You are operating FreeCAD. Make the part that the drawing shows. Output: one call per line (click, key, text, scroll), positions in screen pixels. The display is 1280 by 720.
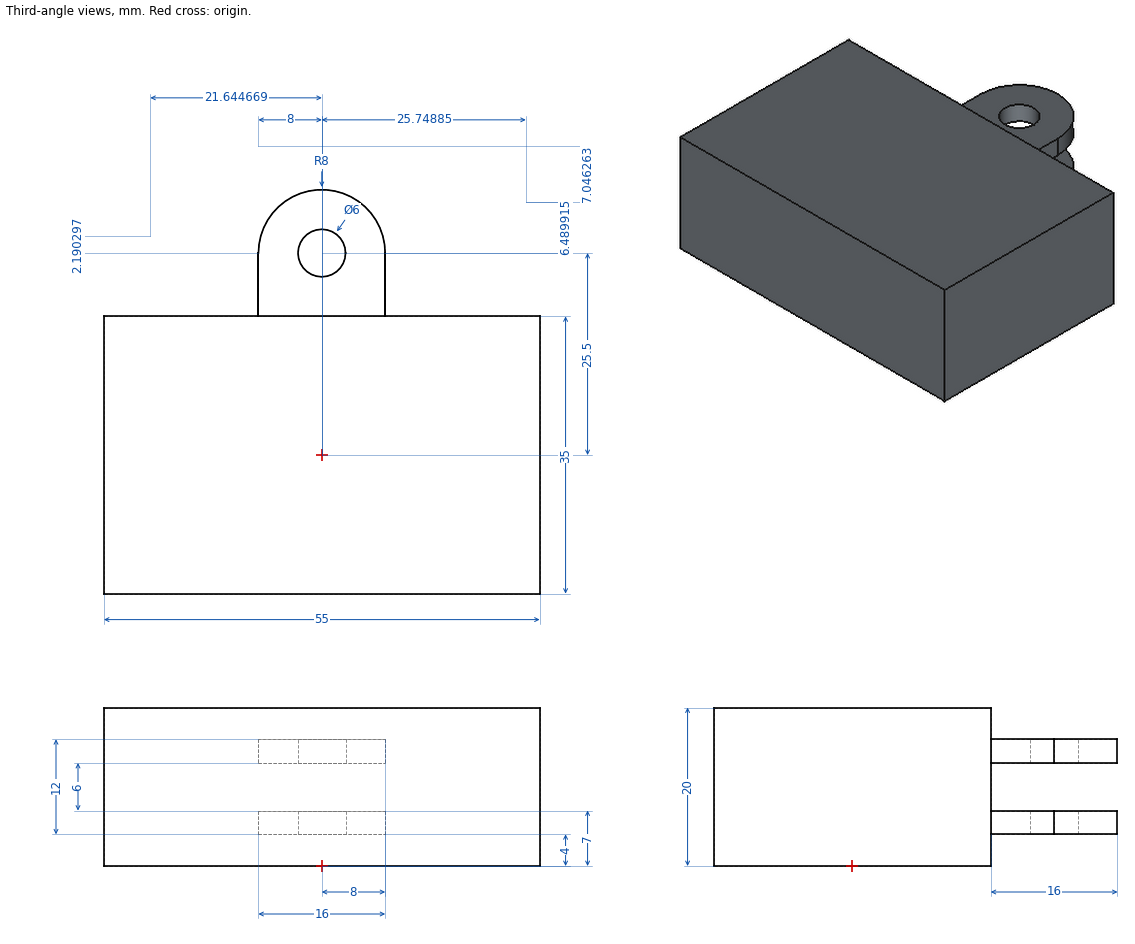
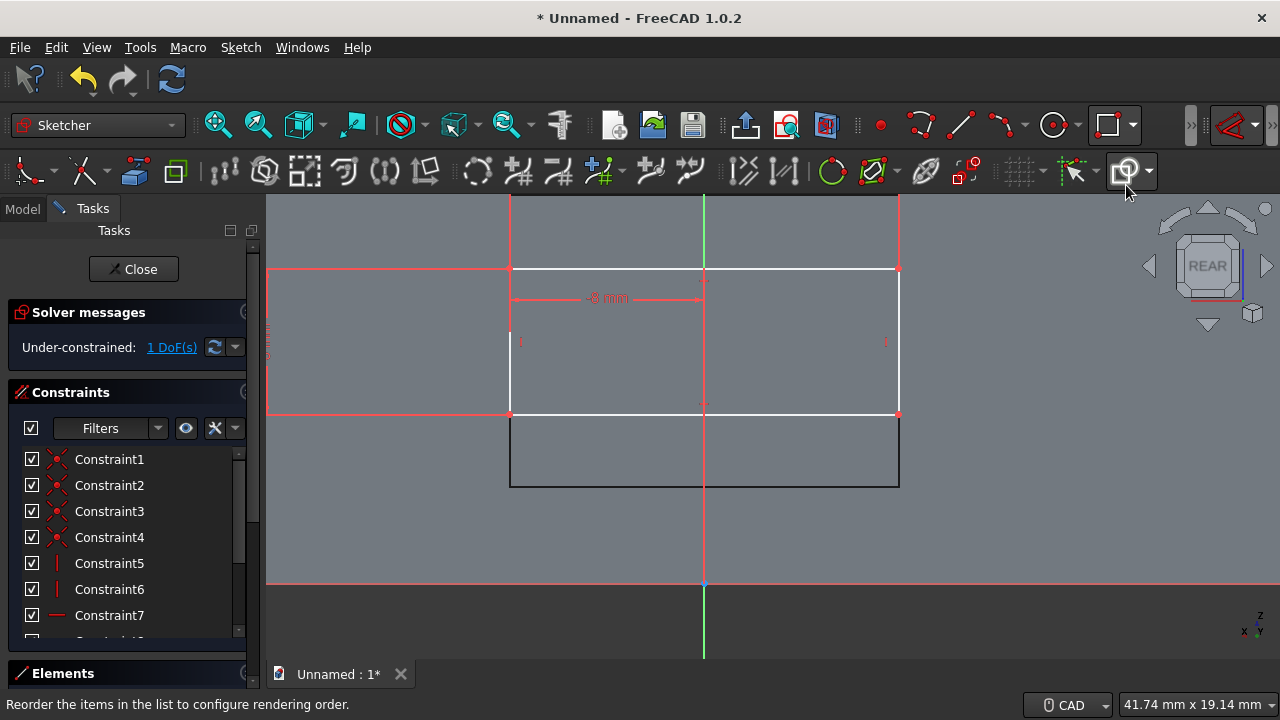
click(510, 415)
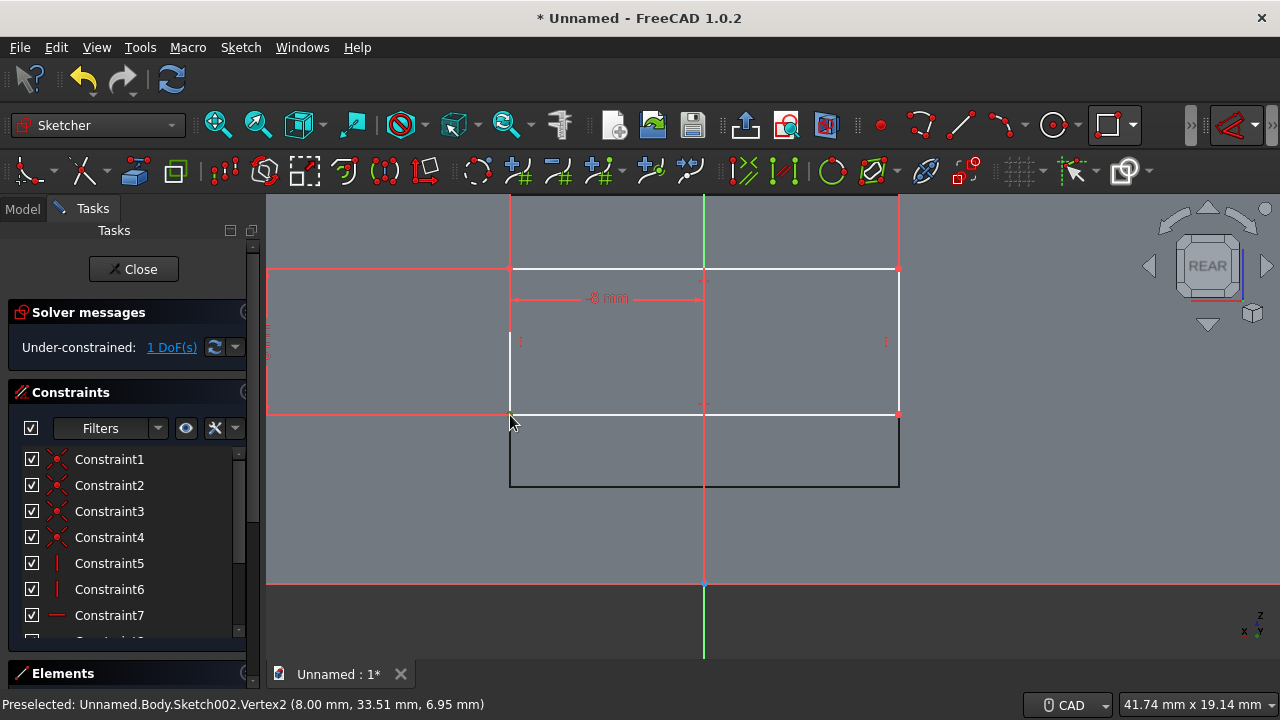
click(1258, 126)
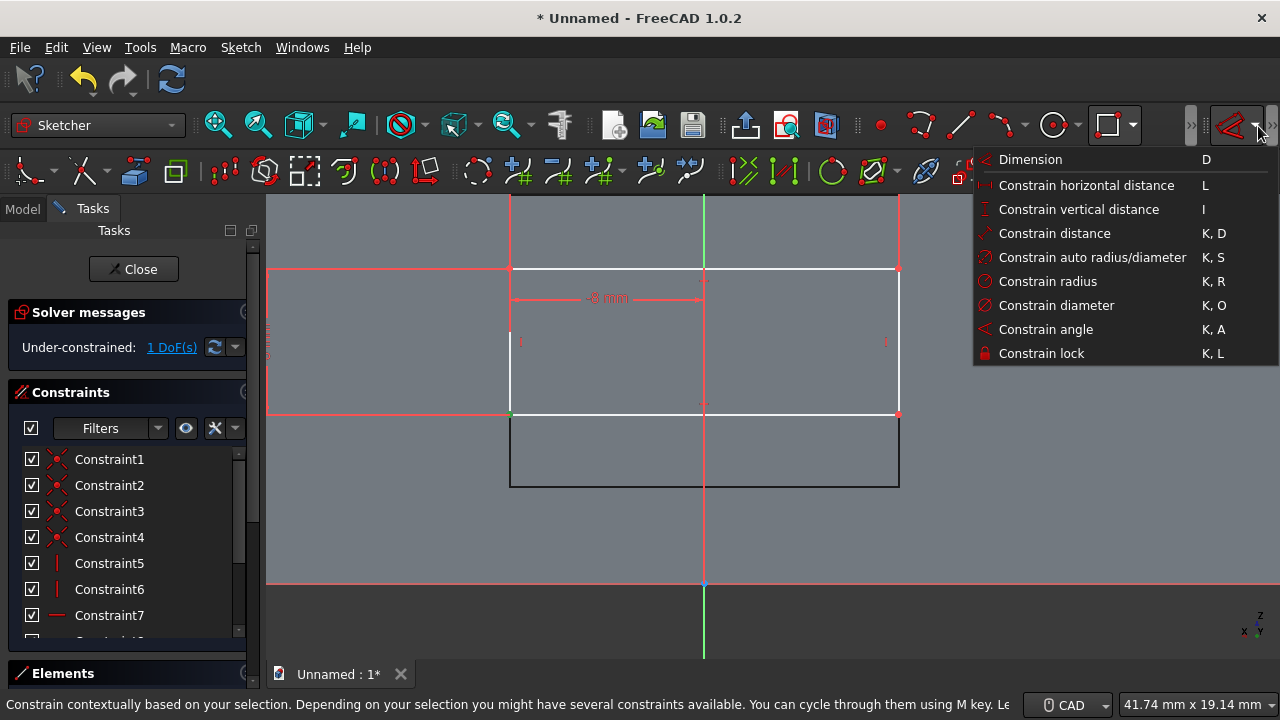
click(1126, 209)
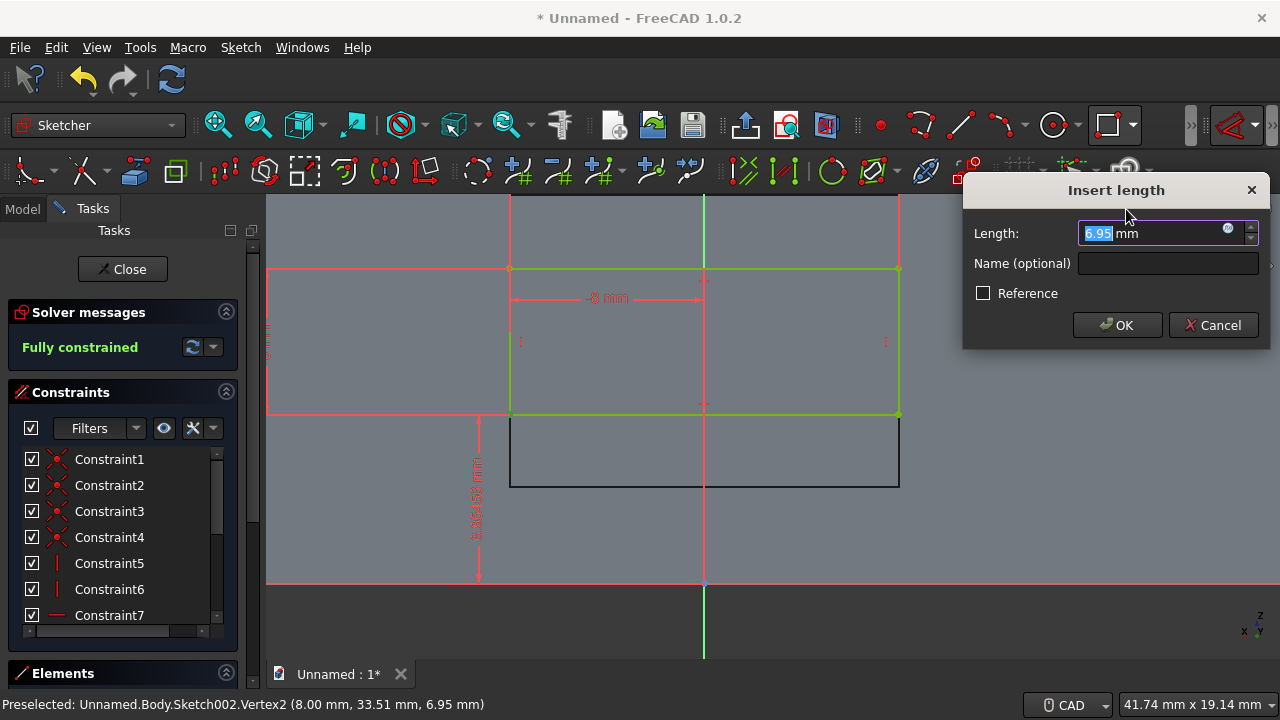
text(7)
key(Return)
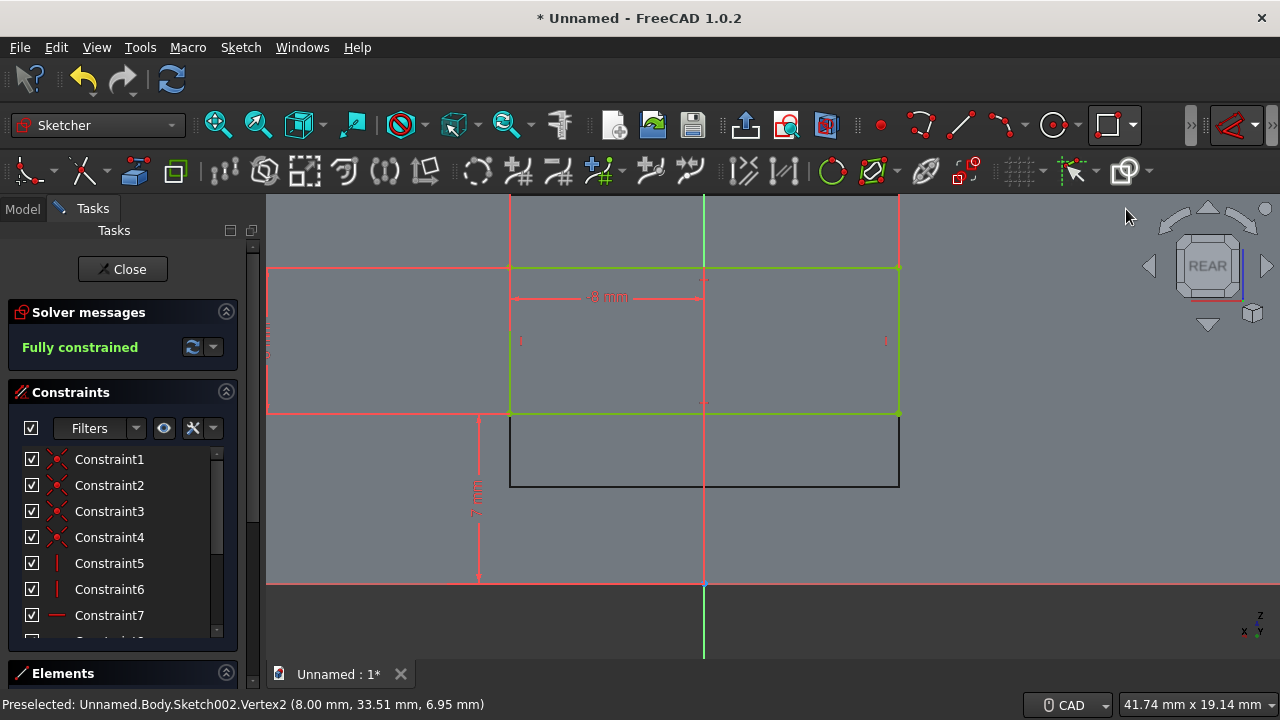
click(123, 269)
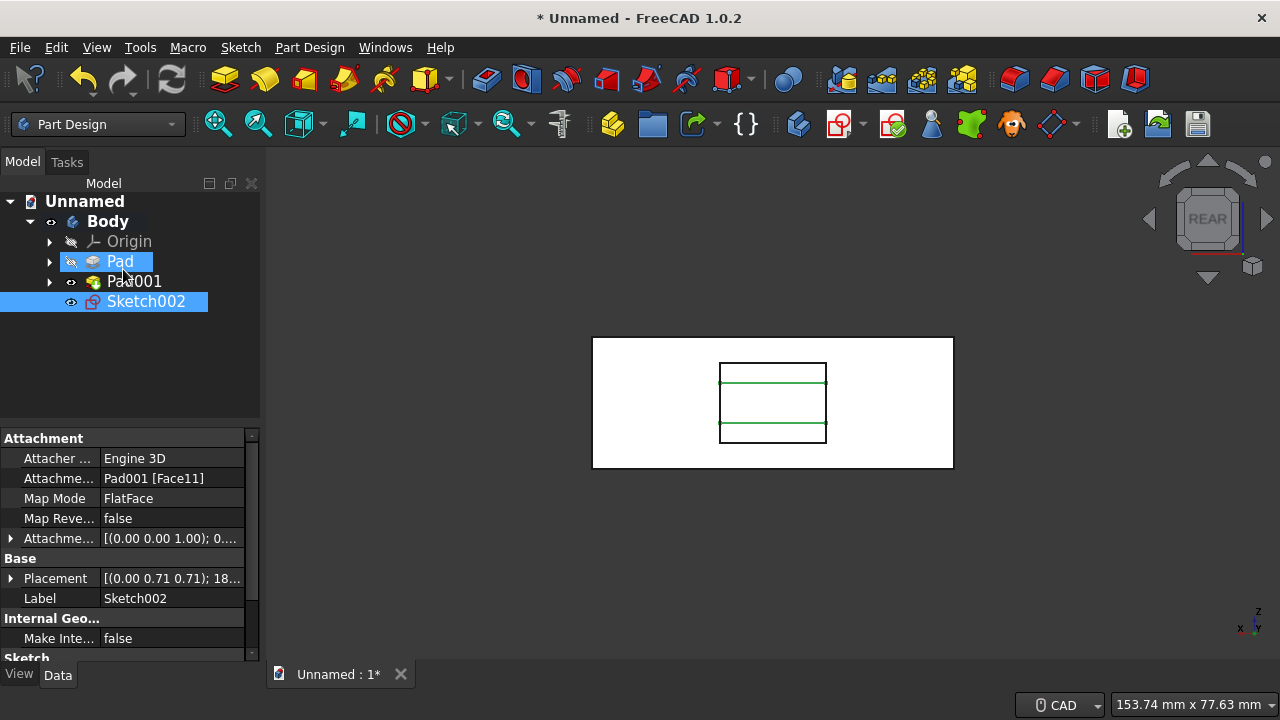
click(488, 80)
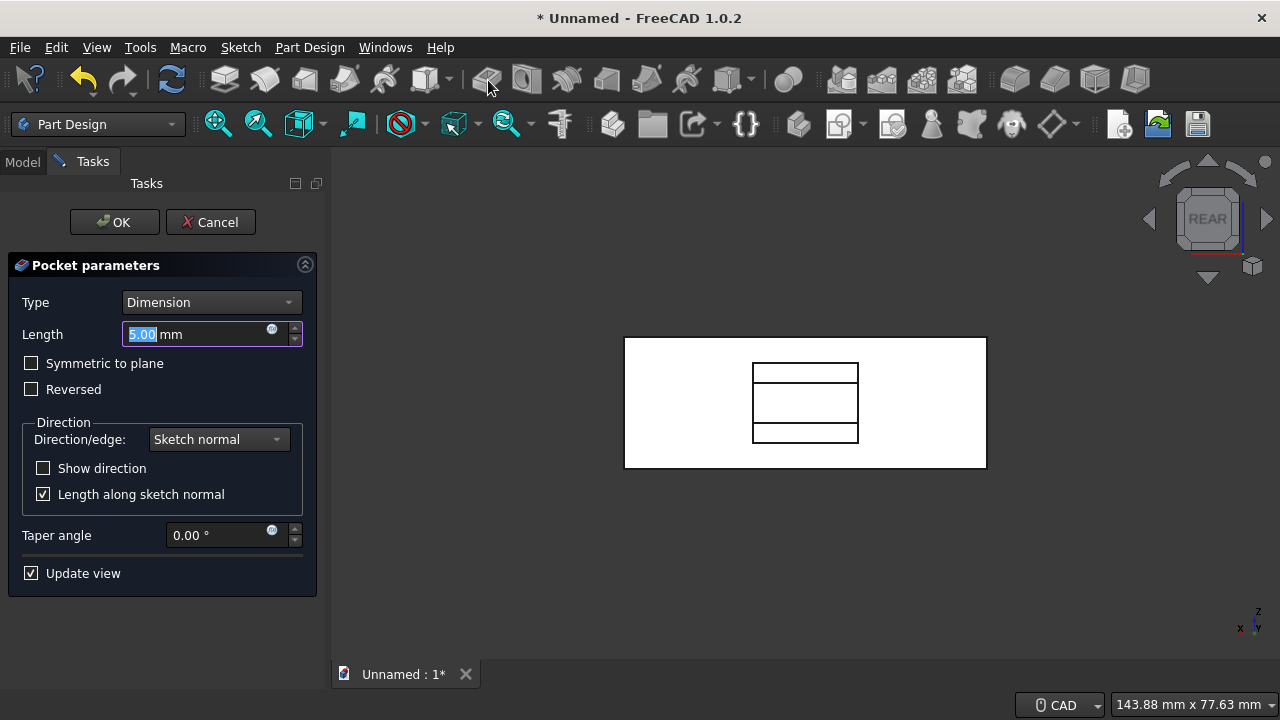
click(212, 302)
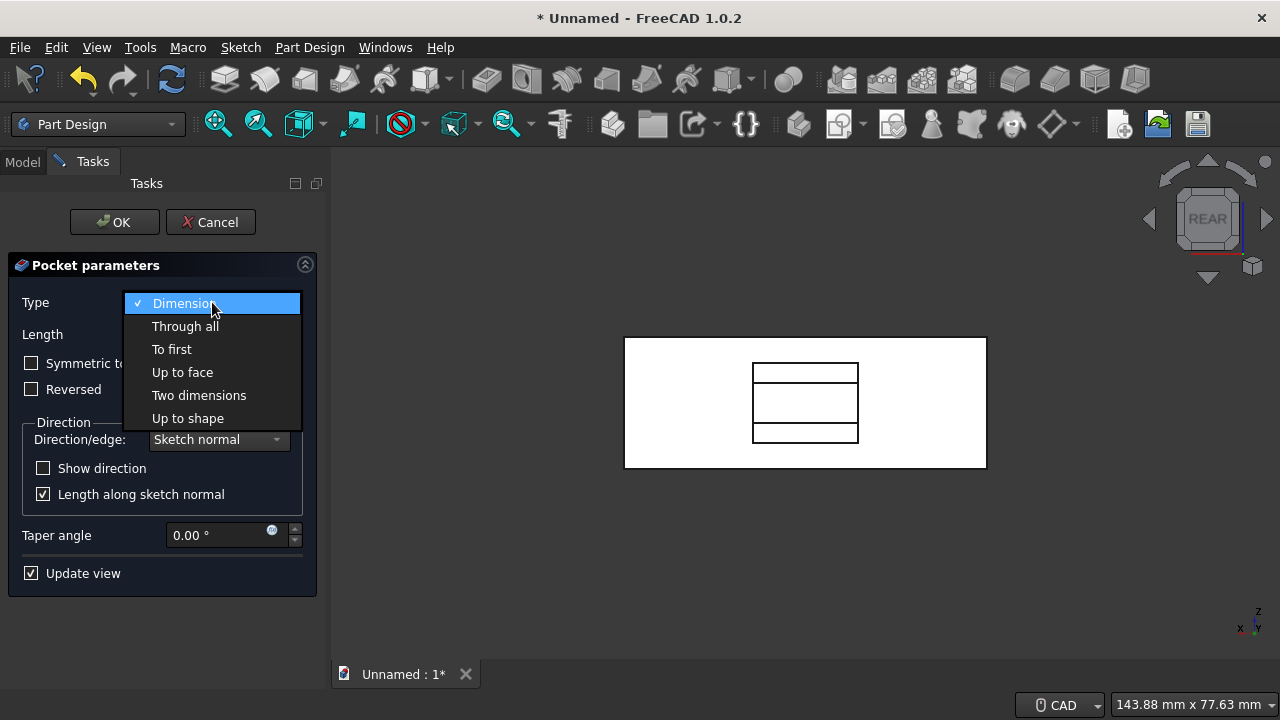
click(212, 396)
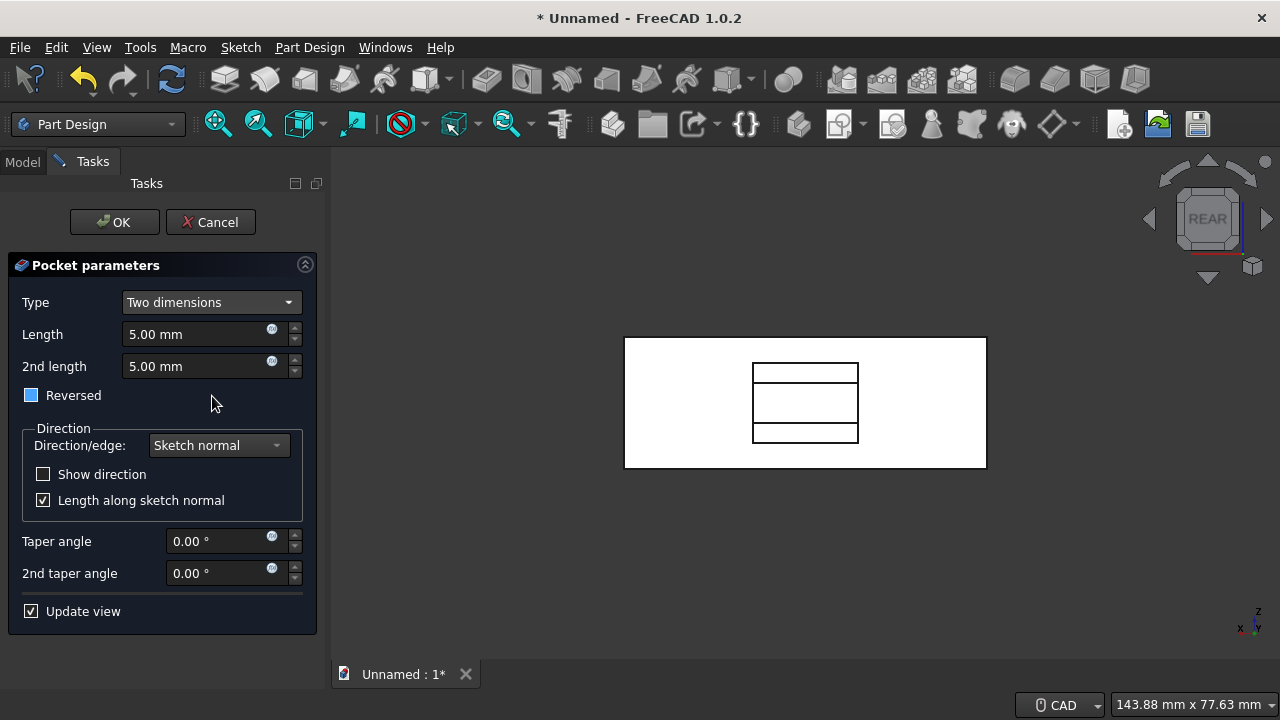
triple_click(204, 334)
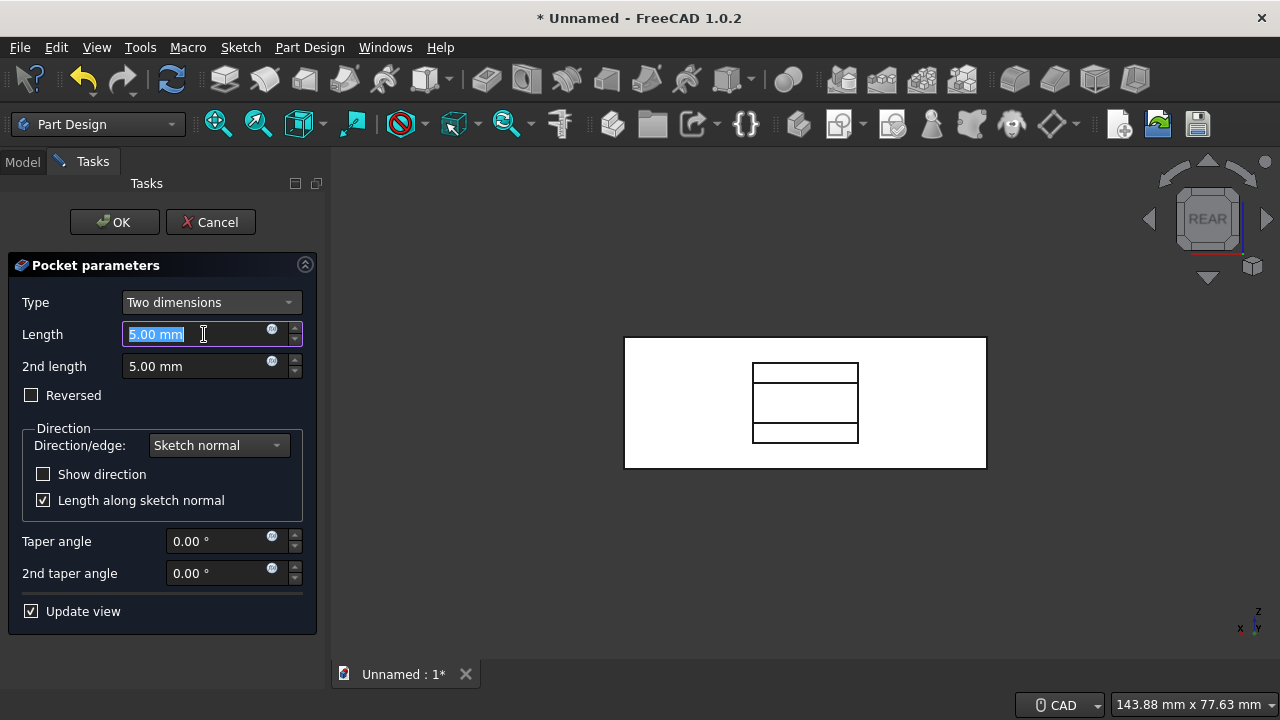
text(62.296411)
key(Tab)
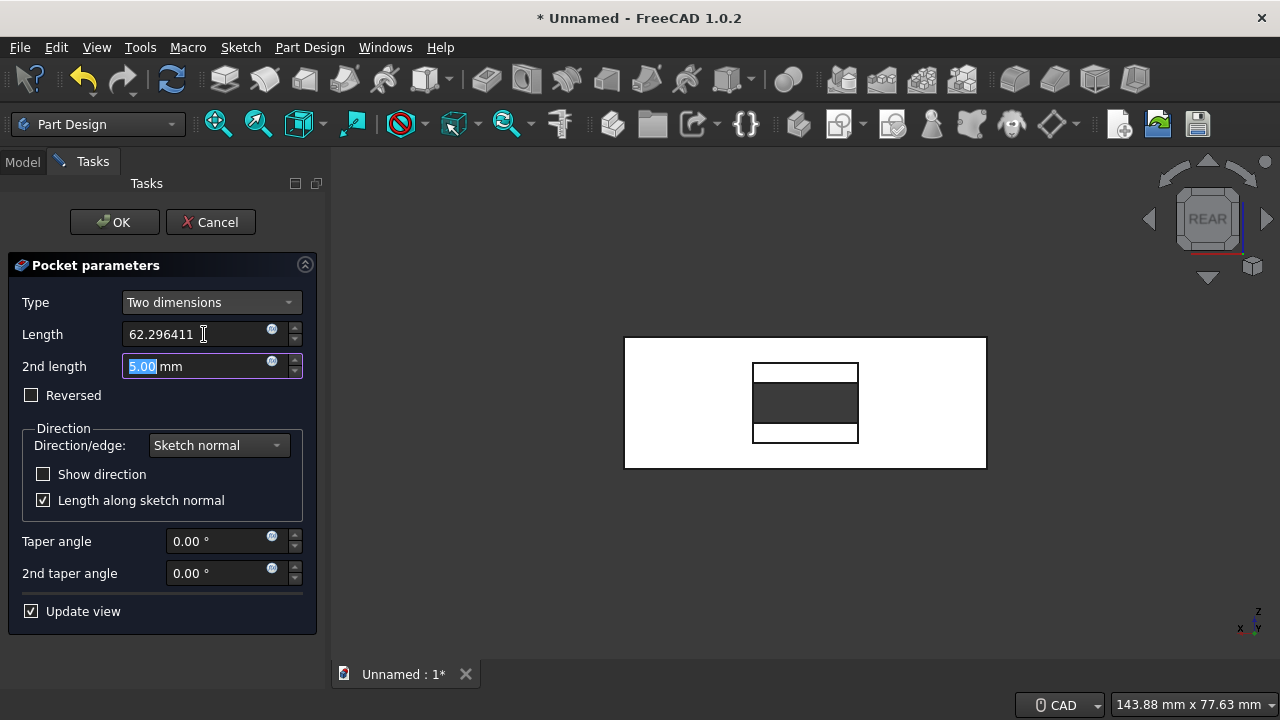
text(16)
key(Tab)